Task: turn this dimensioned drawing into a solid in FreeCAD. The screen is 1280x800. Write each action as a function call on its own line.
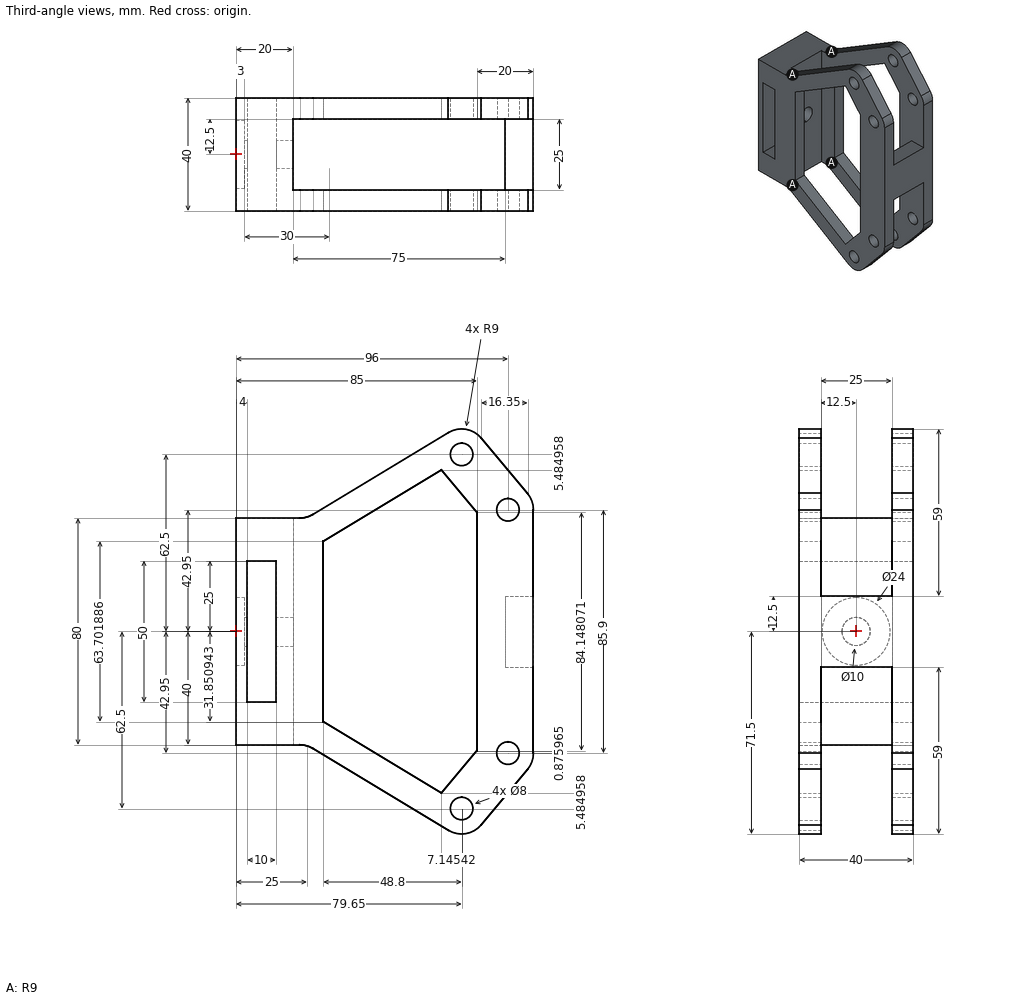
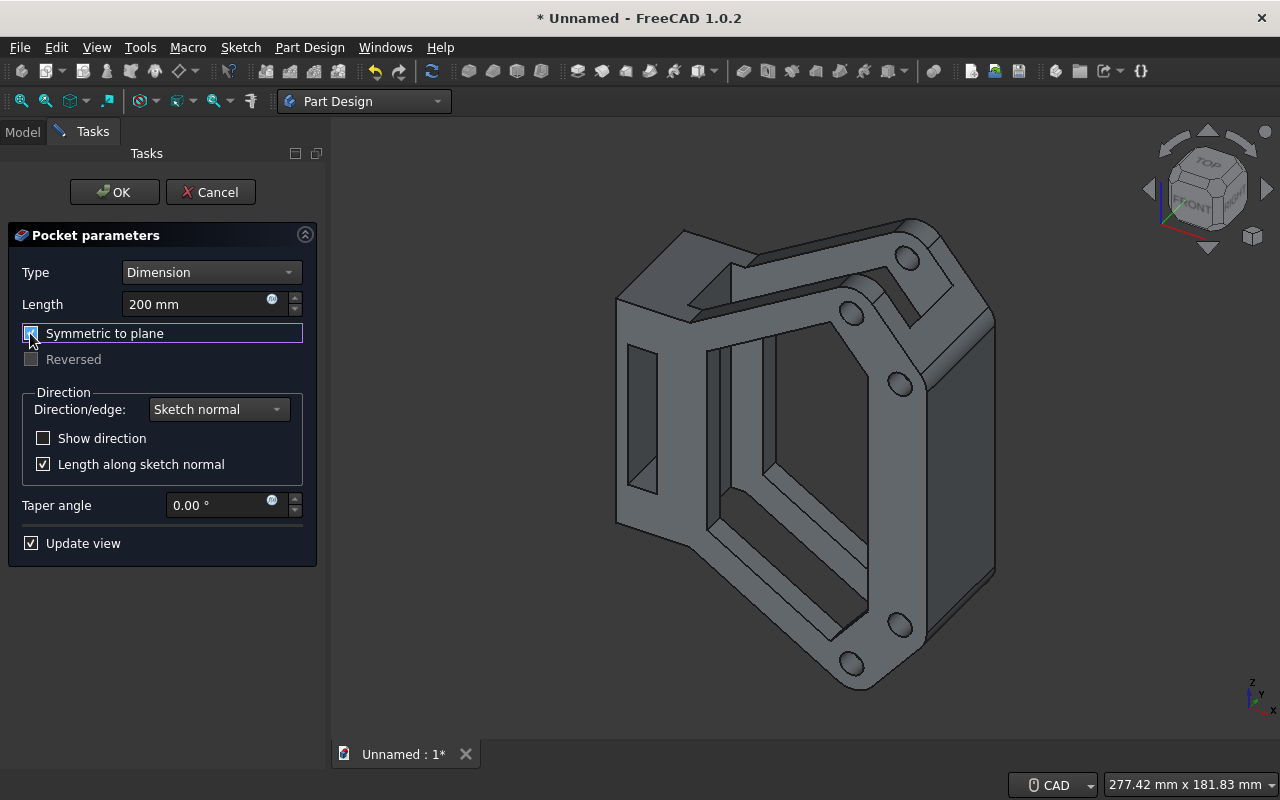
click(115, 192)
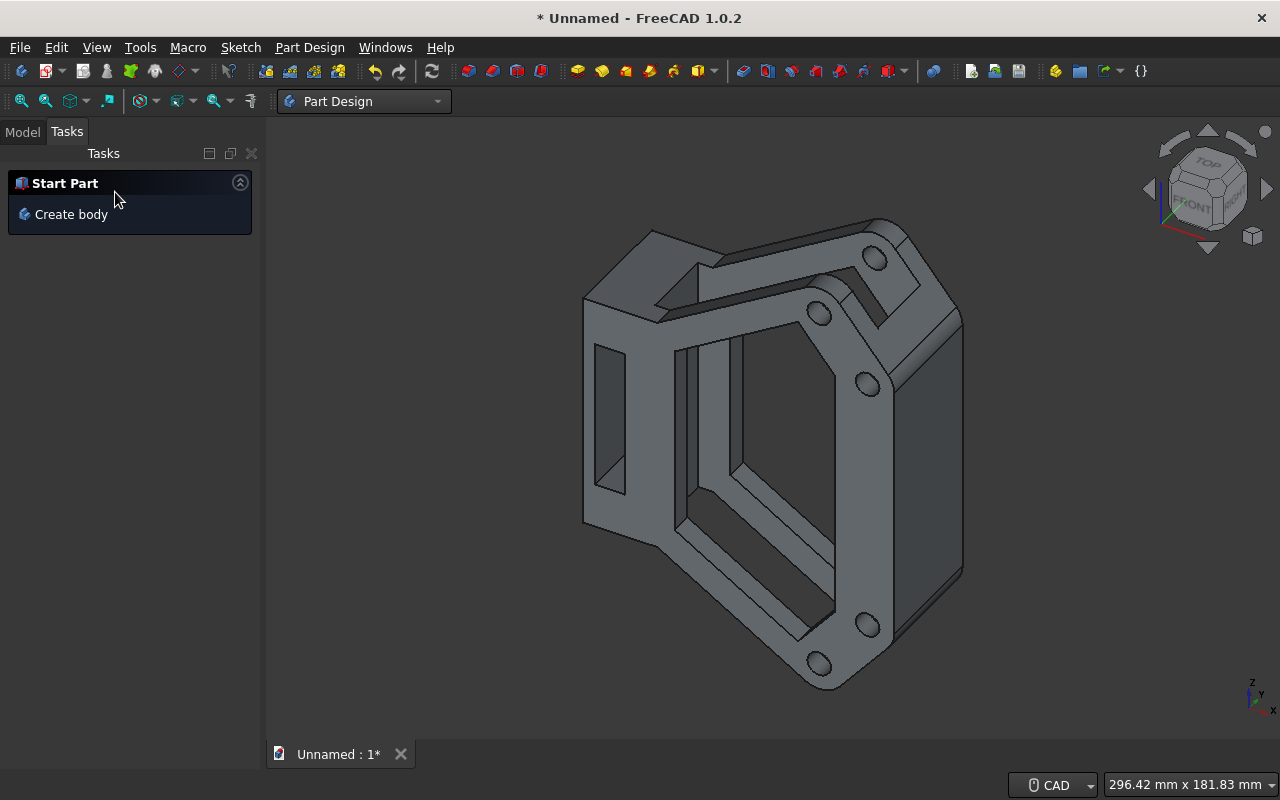
click(929, 479)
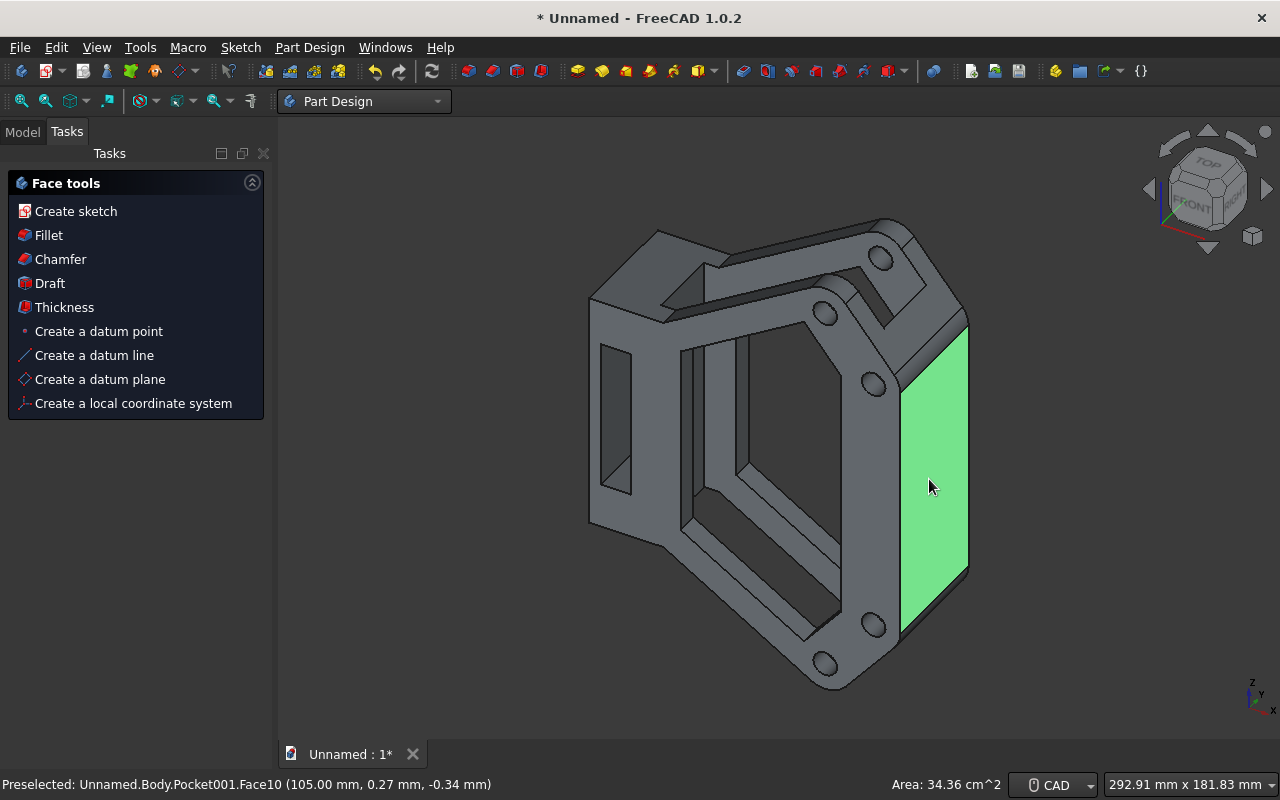
click(46, 72)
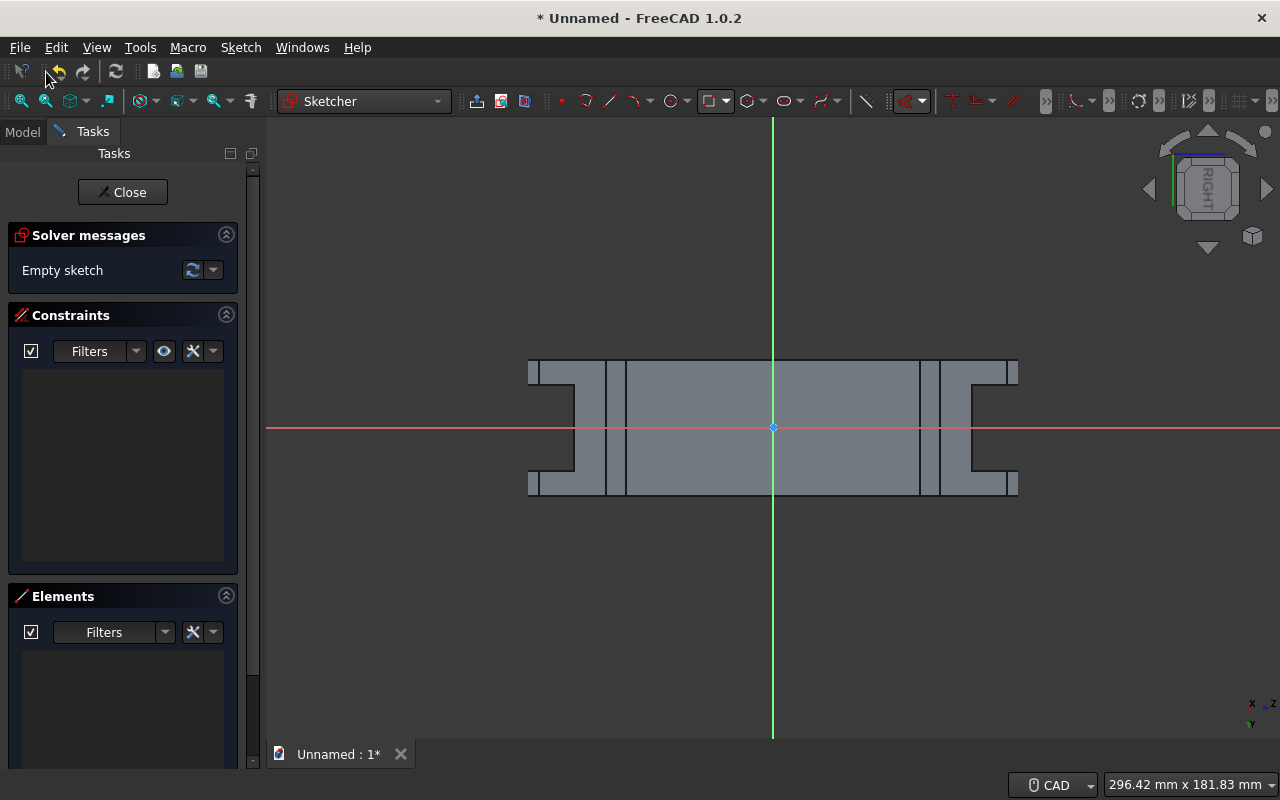
key(g)
key(r)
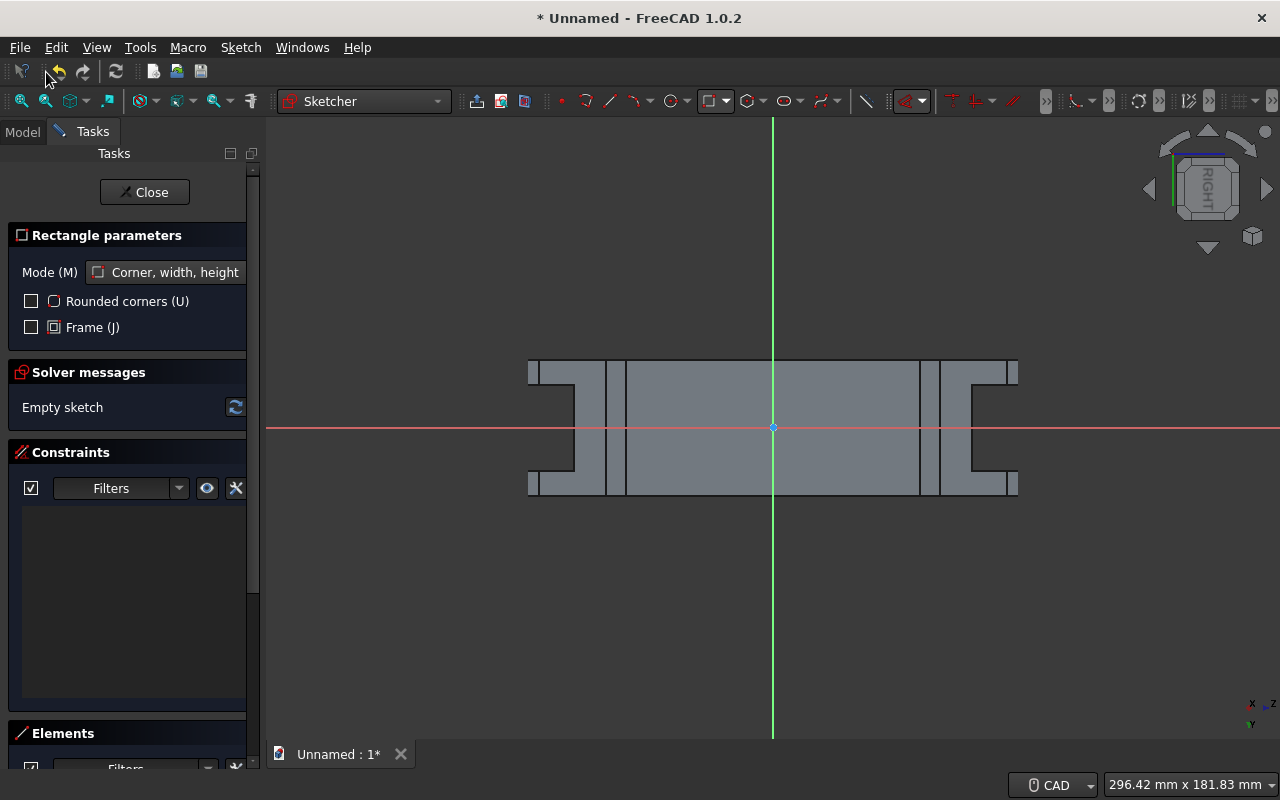
click(816, 385)
move(1018, 471)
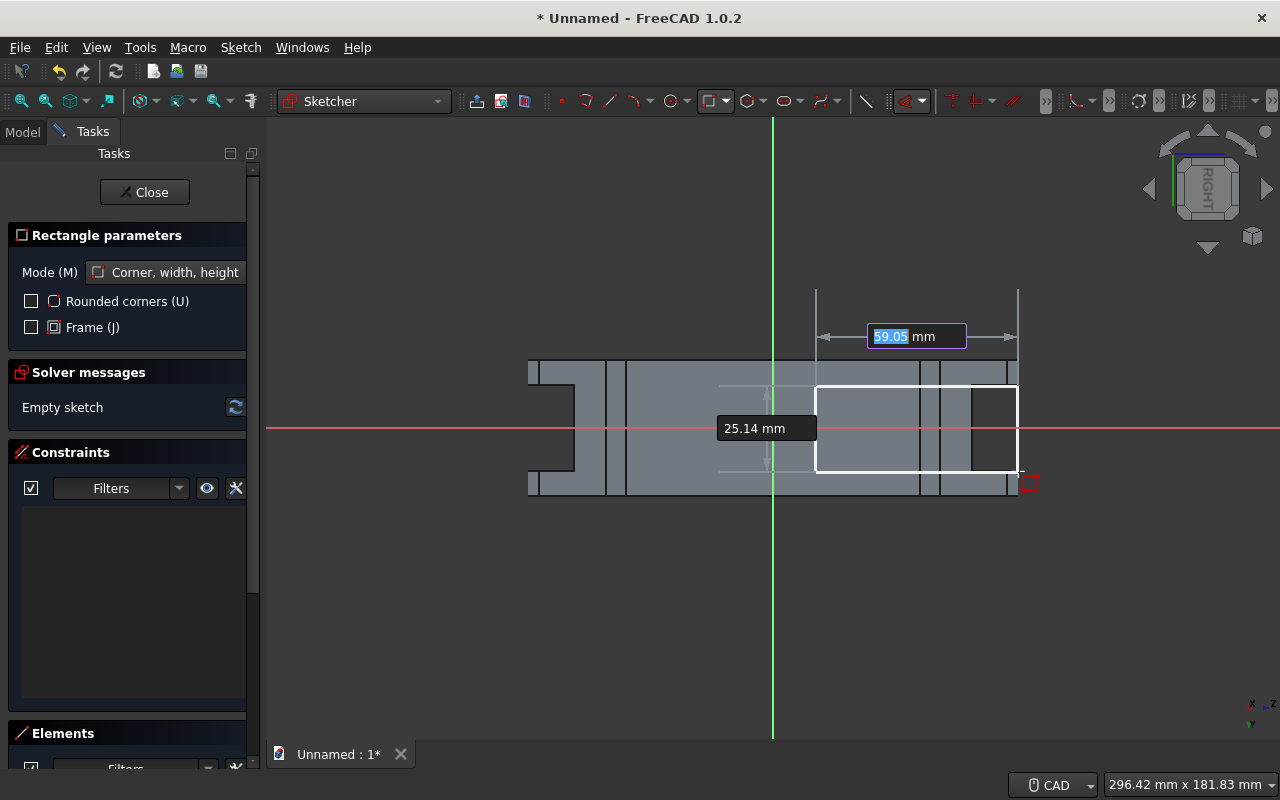
text(59)
key(Tab)
text(25)
key(Return)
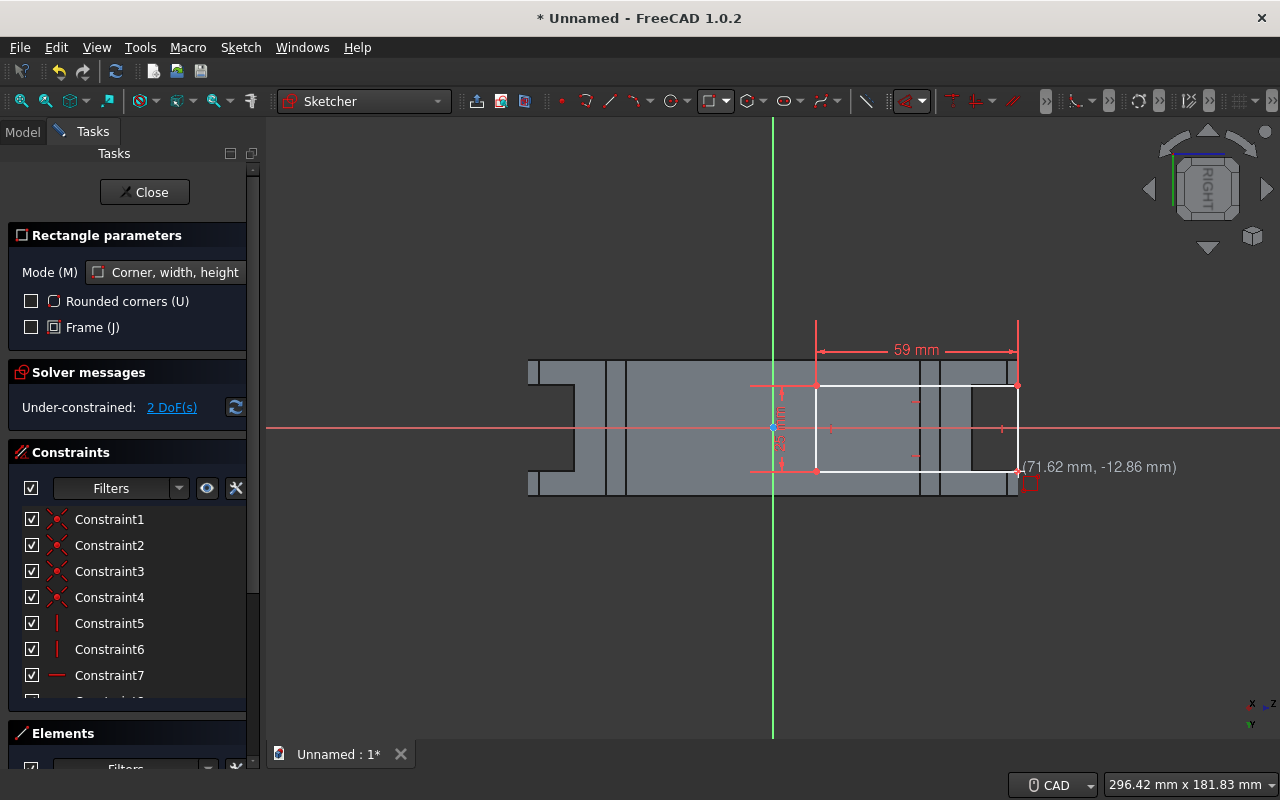
click(528, 385)
move(730, 471)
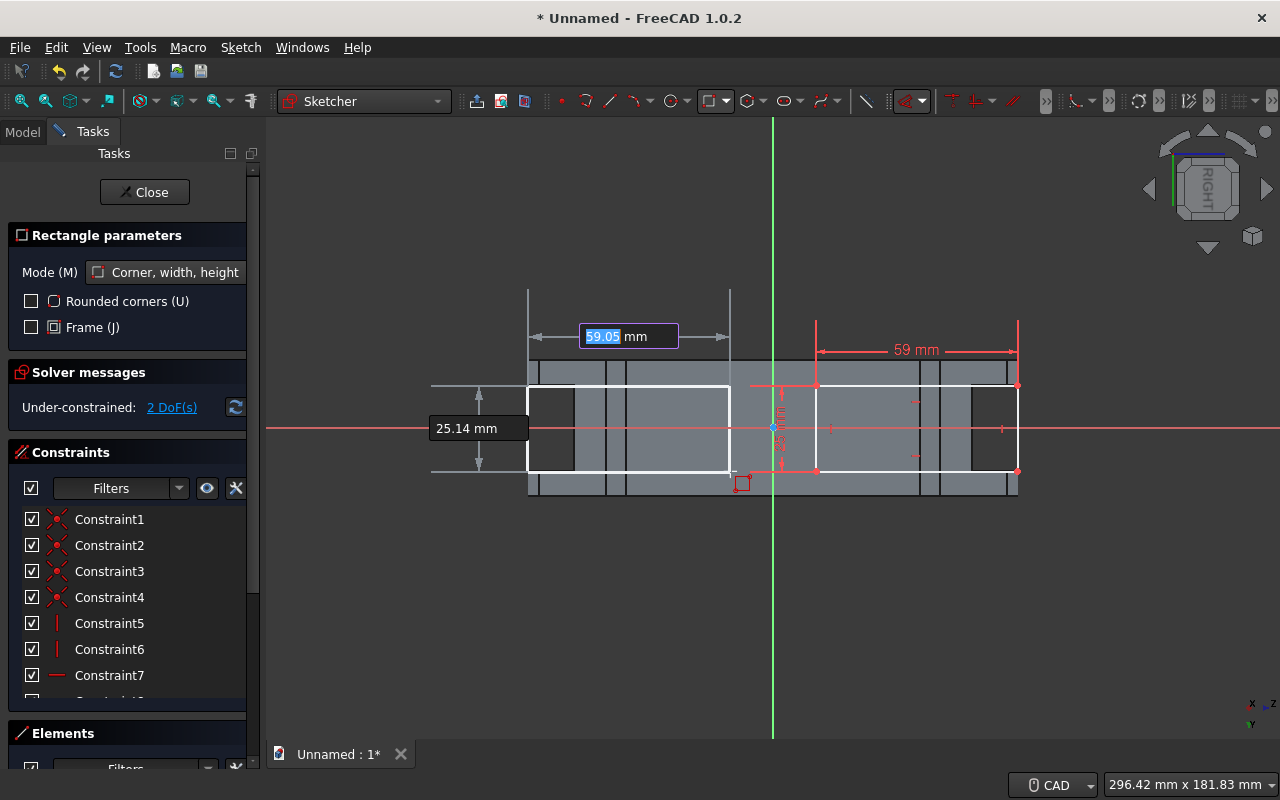
text(59)
key(Tab)
text(25)
key(Return)
key(Escape)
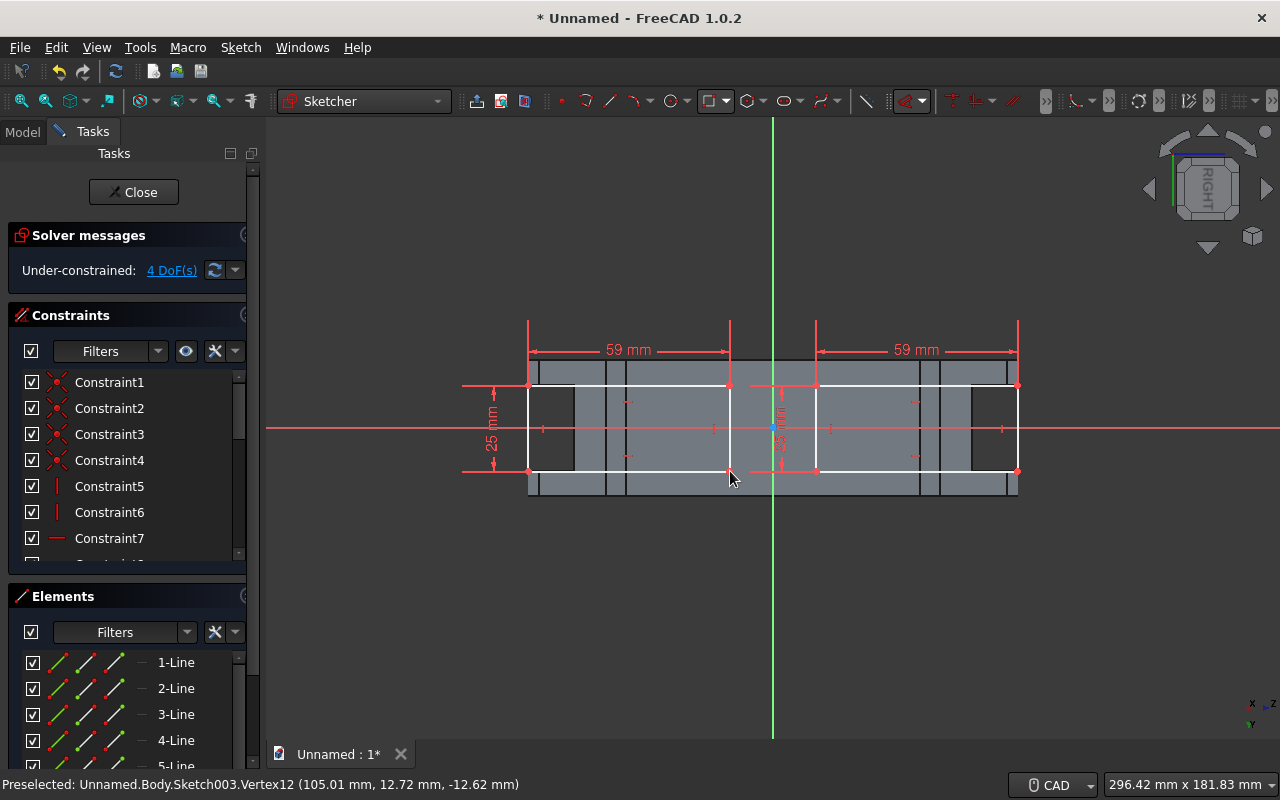
click(816, 386)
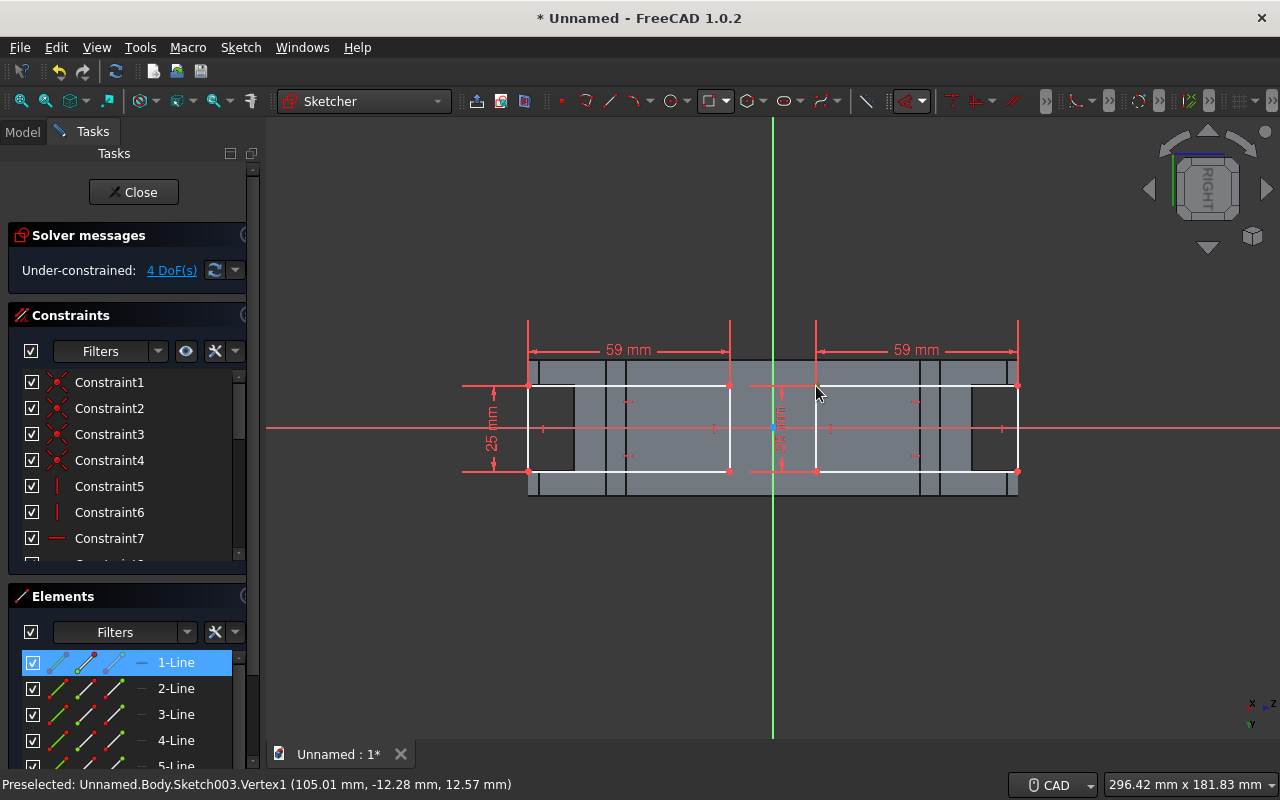
key(l)